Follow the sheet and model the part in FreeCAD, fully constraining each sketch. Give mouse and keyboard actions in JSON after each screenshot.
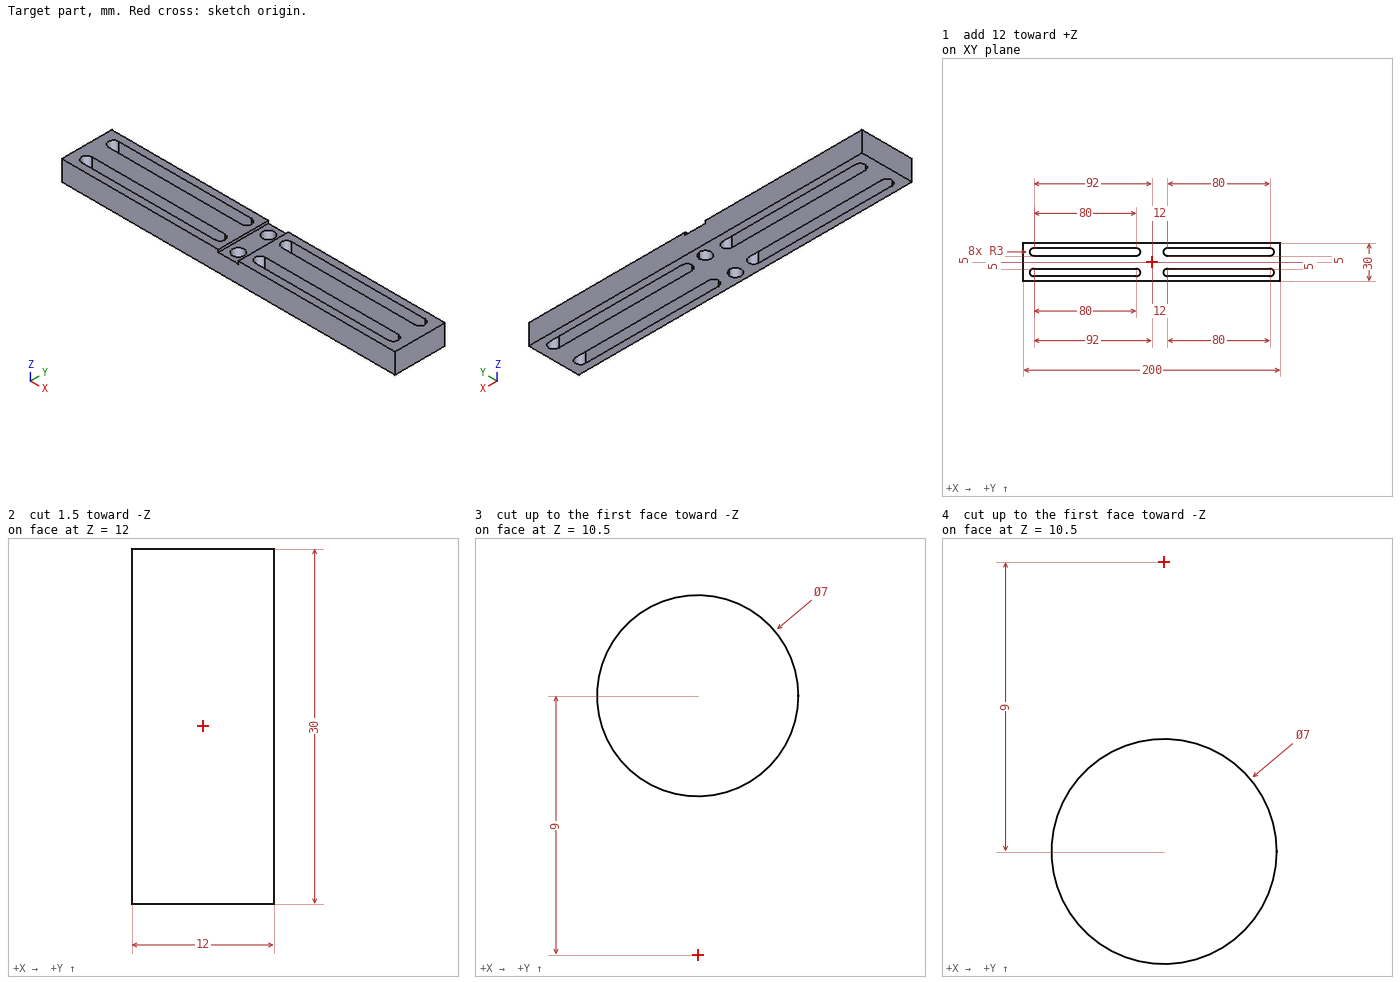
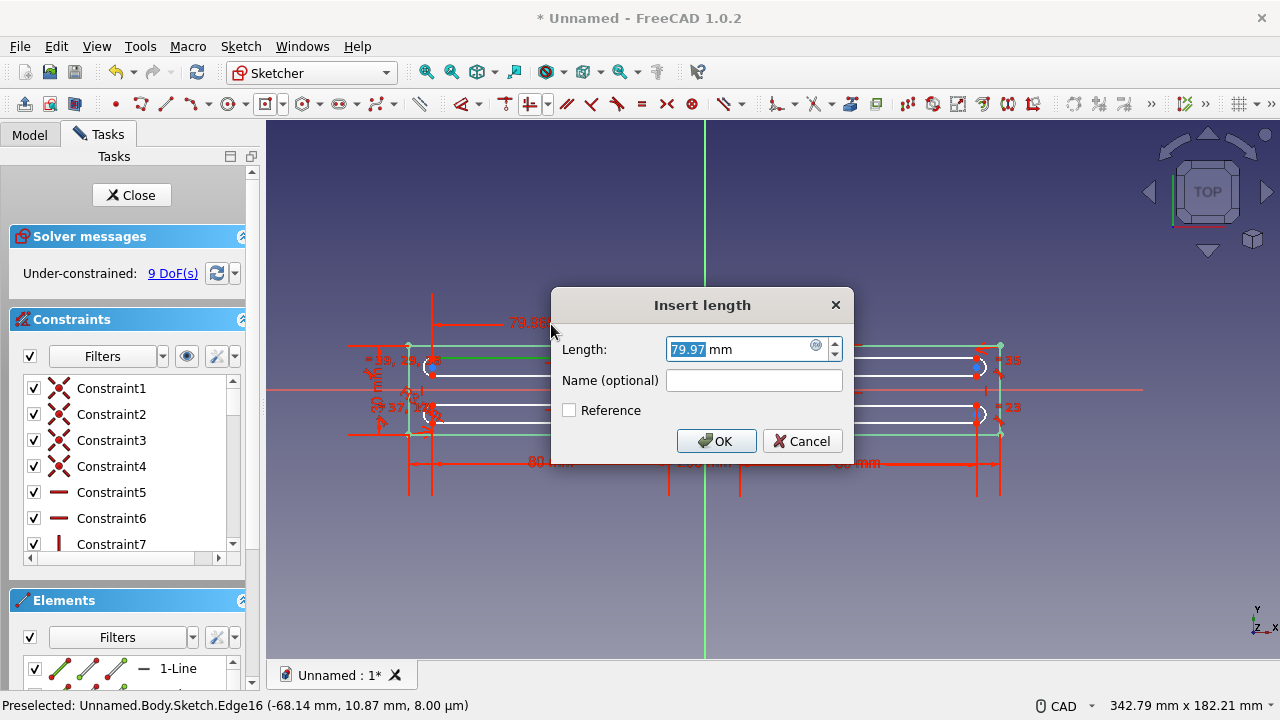
{"action": "type", "text": "80"}
{"action": "key", "text": "Return"}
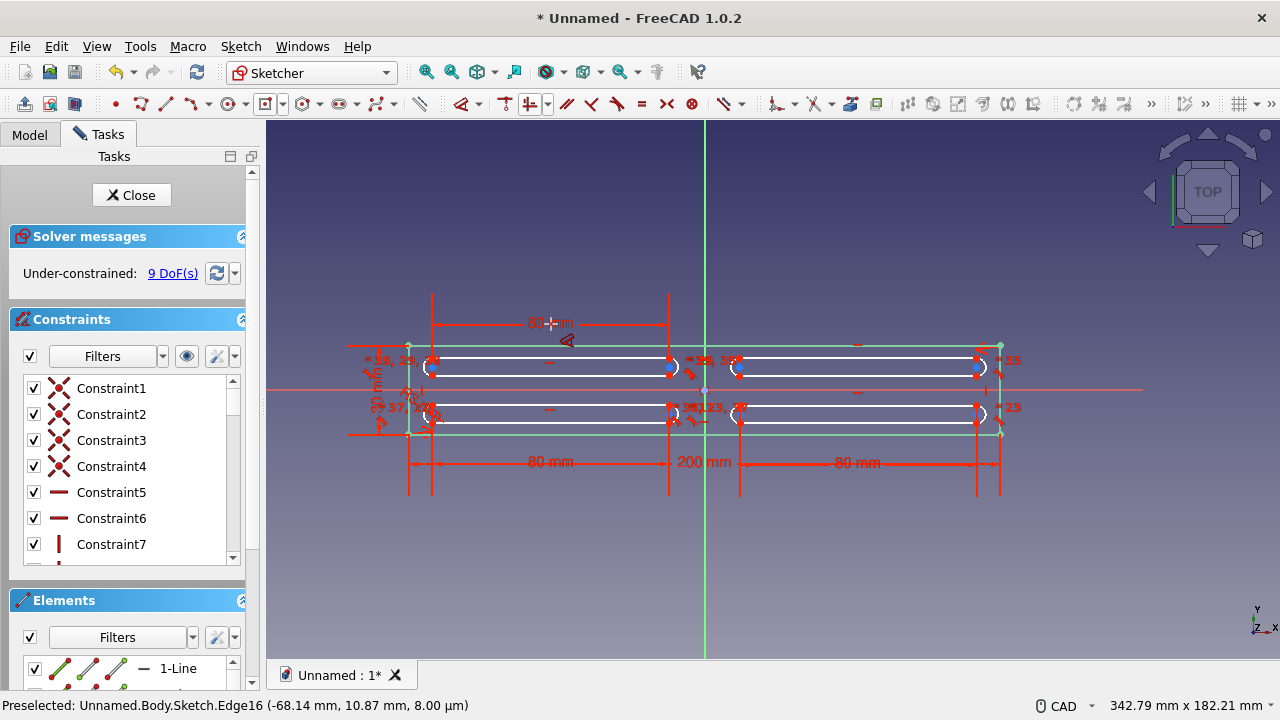
{"action": "left_click", "coordinate": [811, 358]}
{"action": "left_click", "coordinate": [858, 324]}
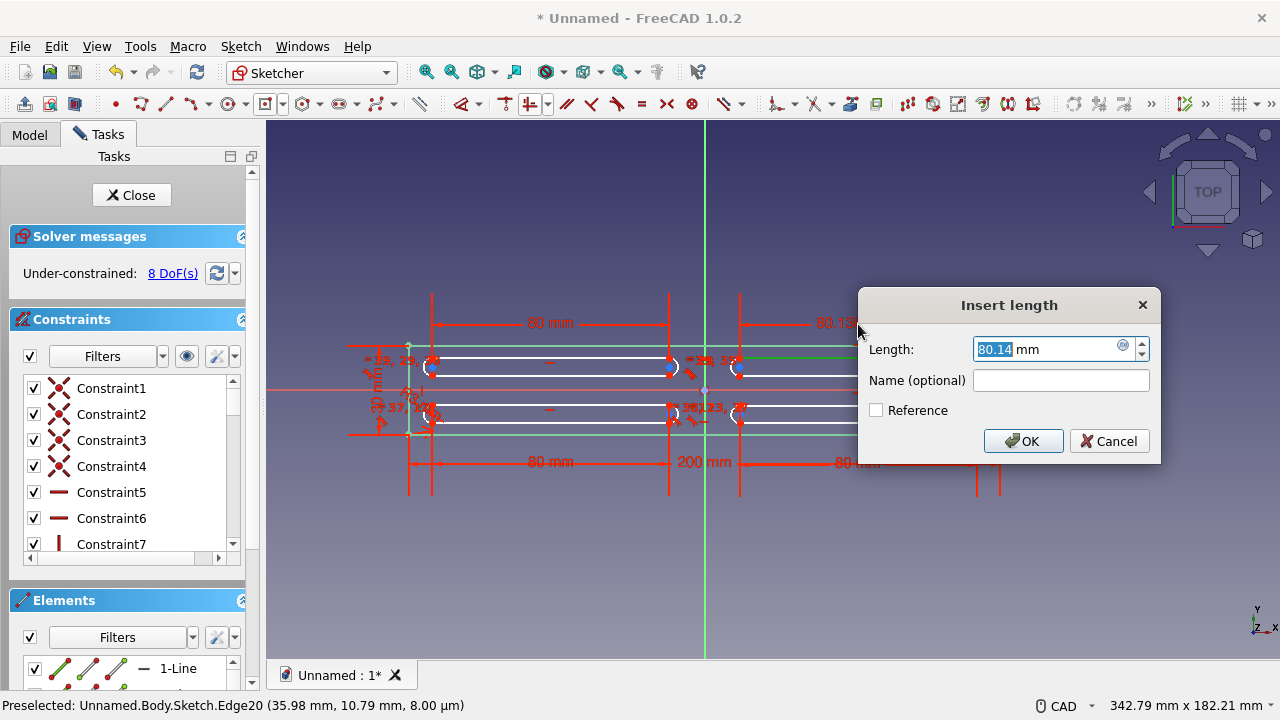
{"action": "type", "text": "80"}
{"action": "key", "text": "Return"}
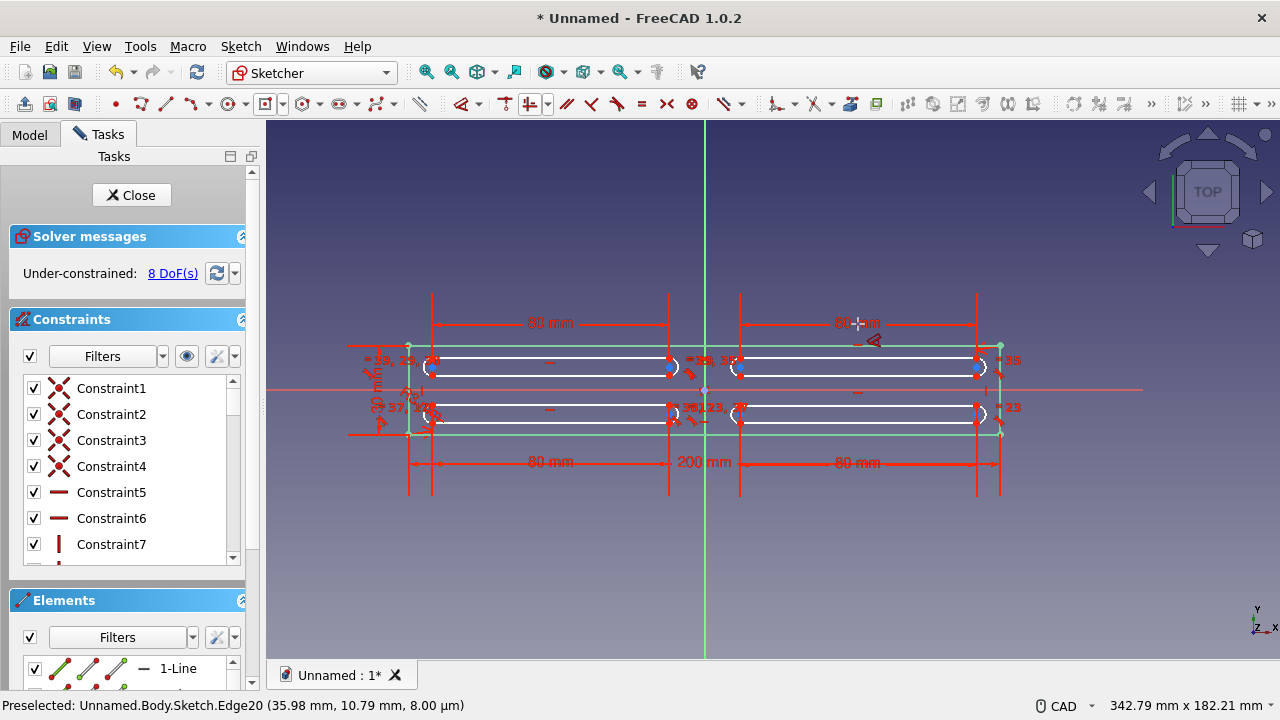
{"action": "scroll", "coordinate": [432, 405], "scroll_direction": "up", "scroll_amount": 5}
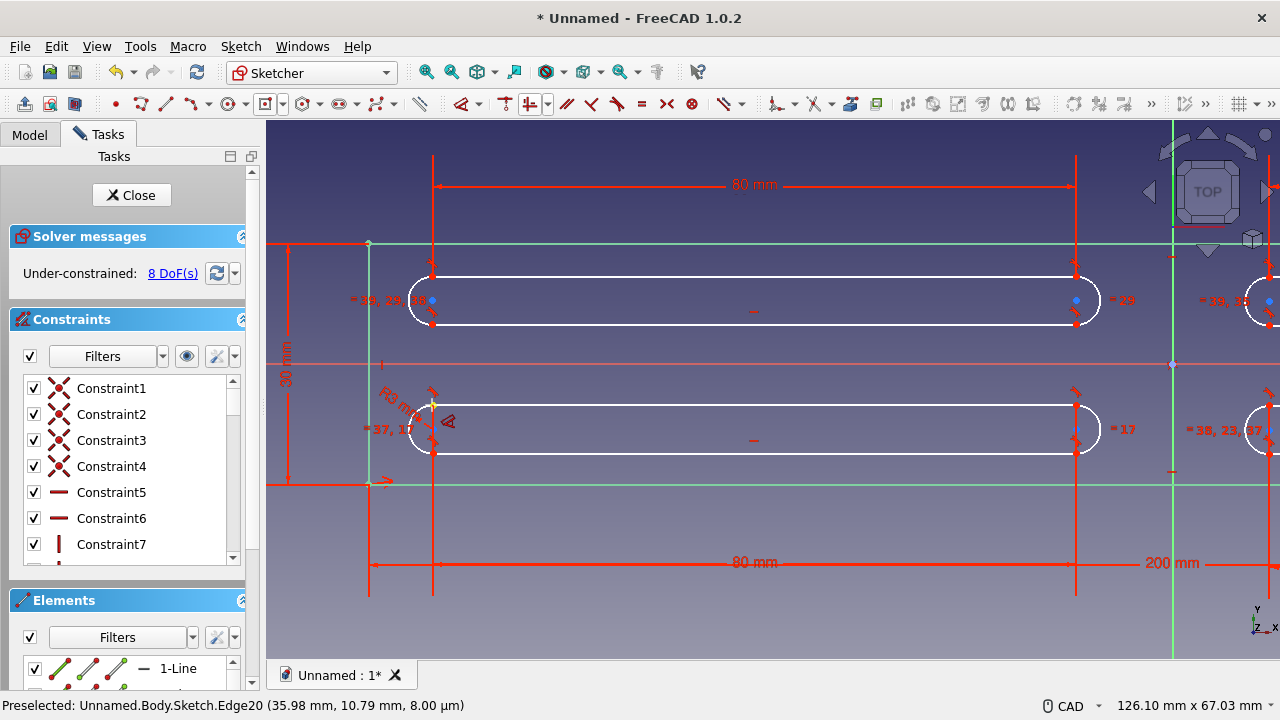
{"action": "left_click", "coordinate": [433, 405]}
{"action": "left_click", "coordinate": [399, 385]}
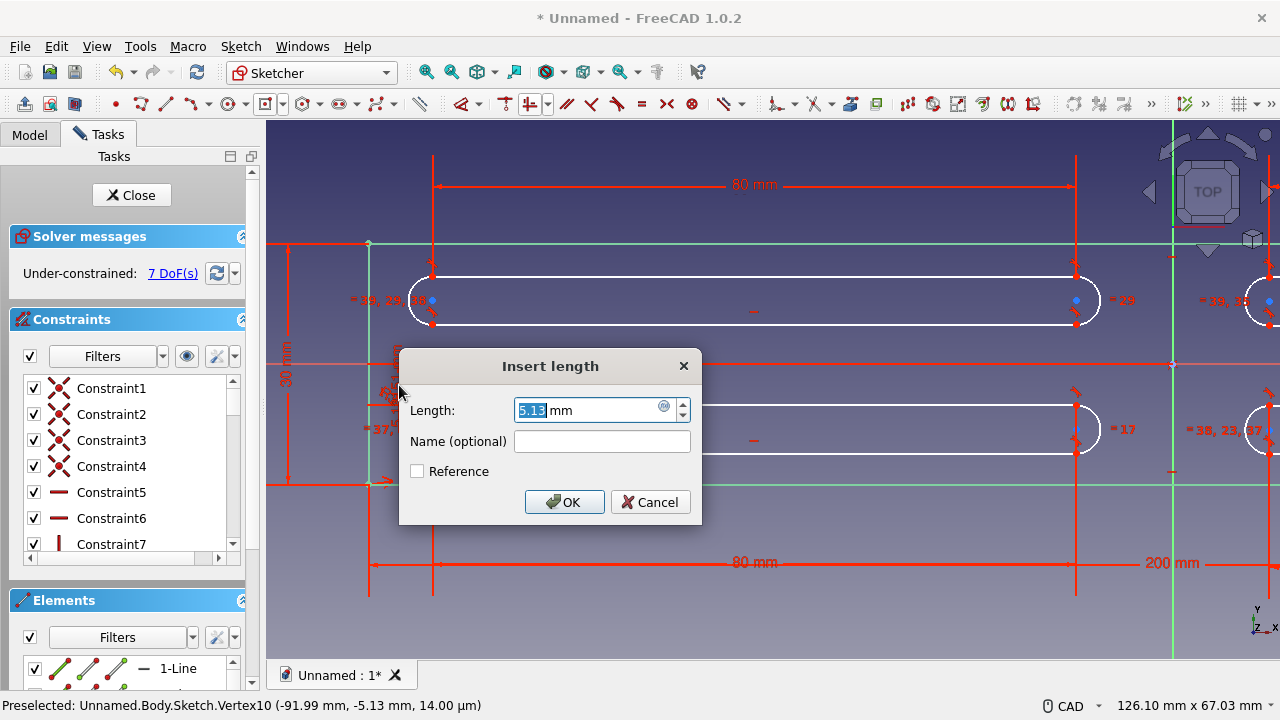
{"action": "type", "text": "5"}
{"action": "key", "text": "Return"}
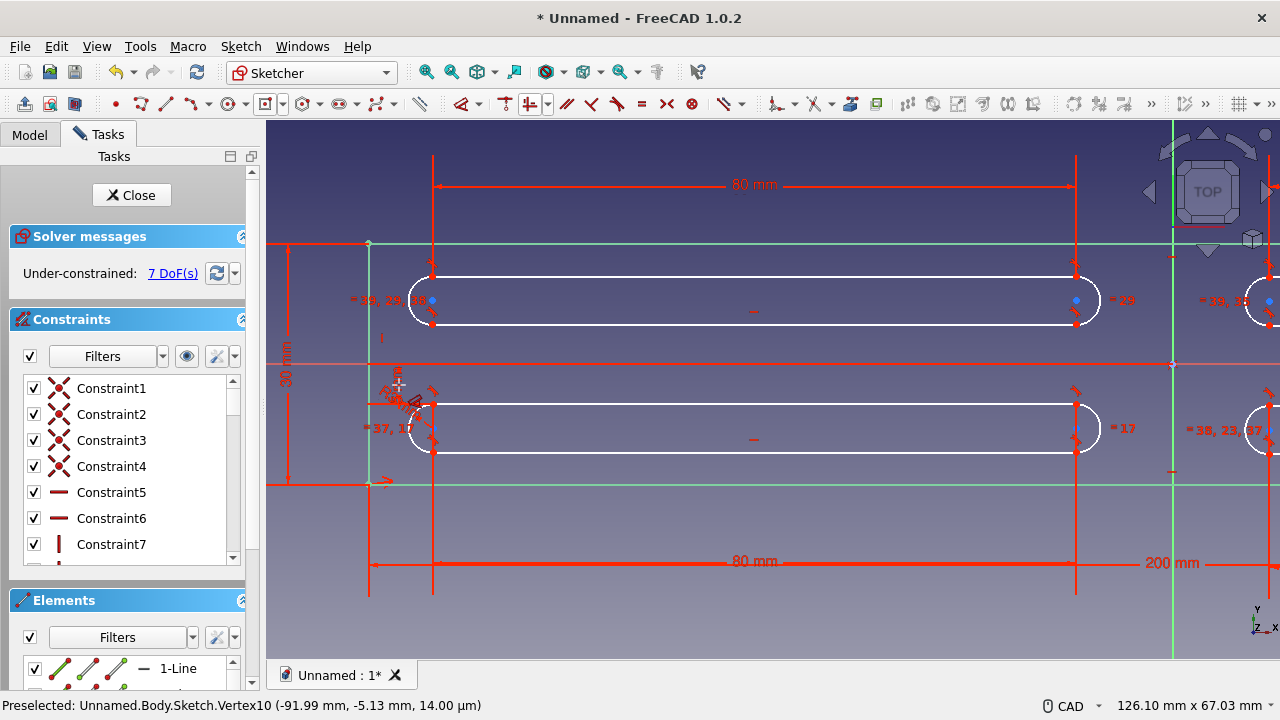
{"action": "scroll", "coordinate": [432, 404], "scroll_direction": "down", "scroll_amount": 5}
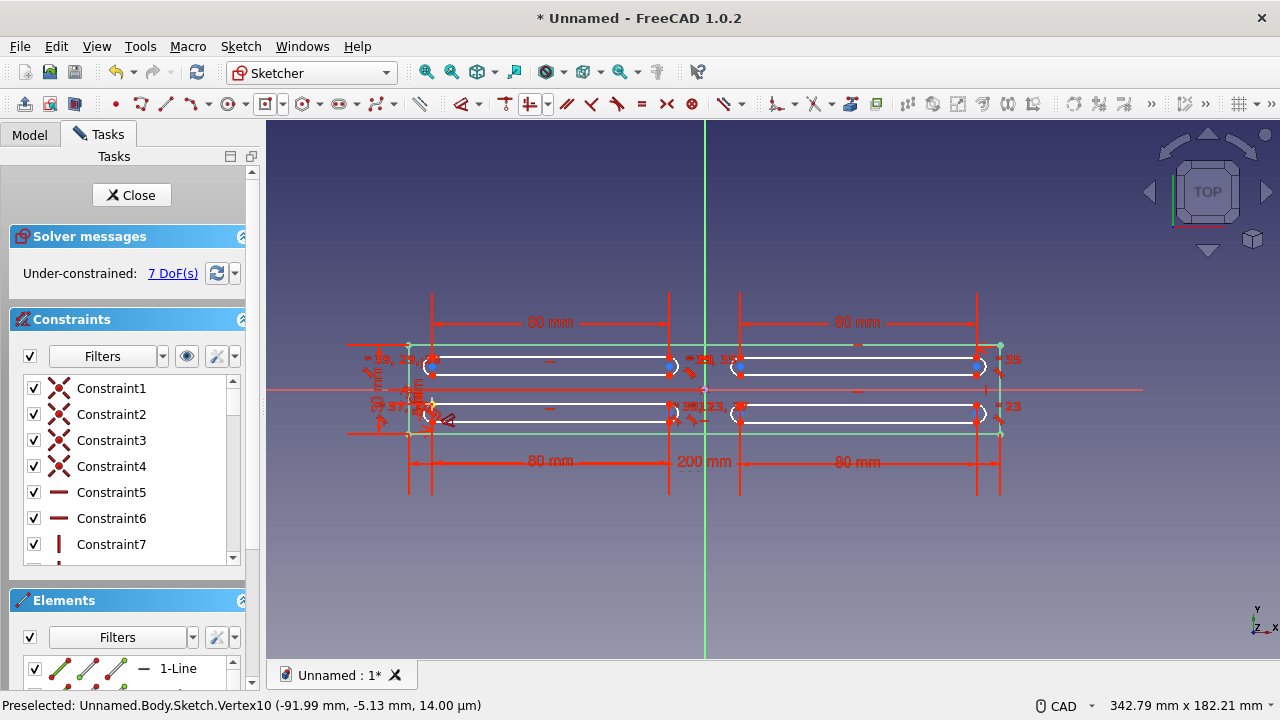
{"action": "scroll", "coordinate": [740, 405], "scroll_direction": "up", "scroll_amount": 5}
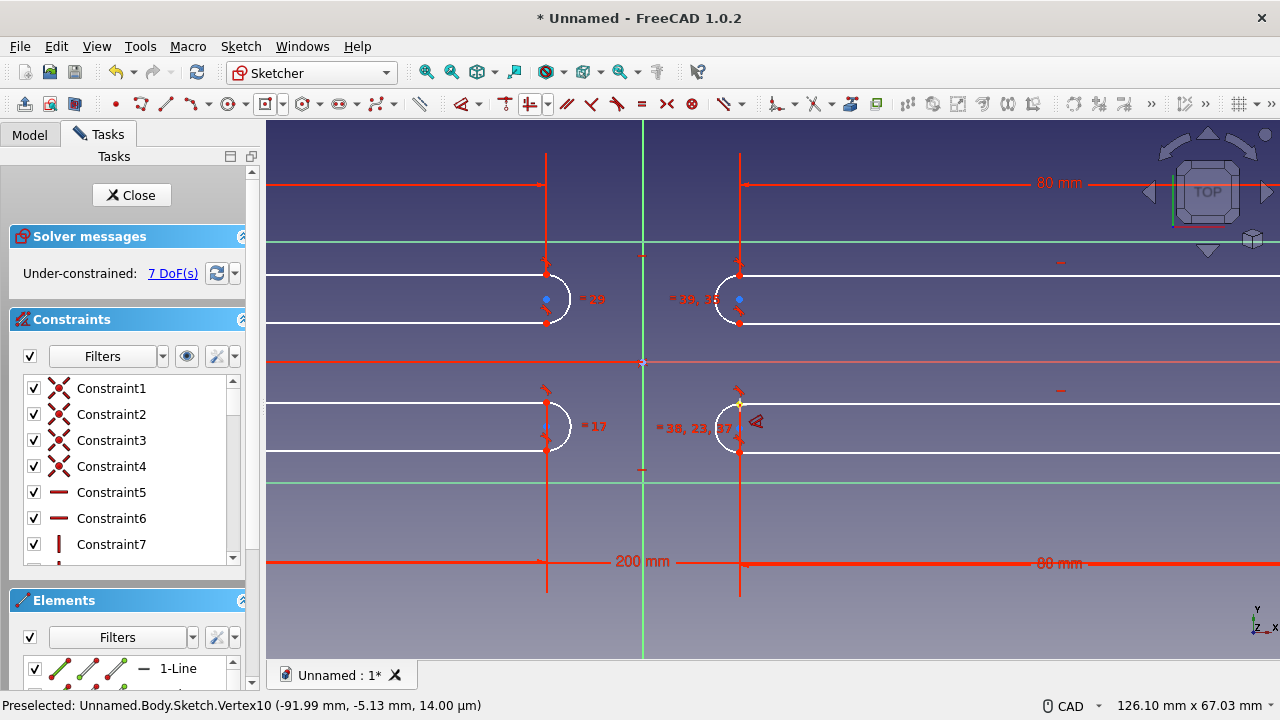
{"action": "left_click", "coordinate": [740, 404]}
{"action": "left_click", "coordinate": [774, 383]}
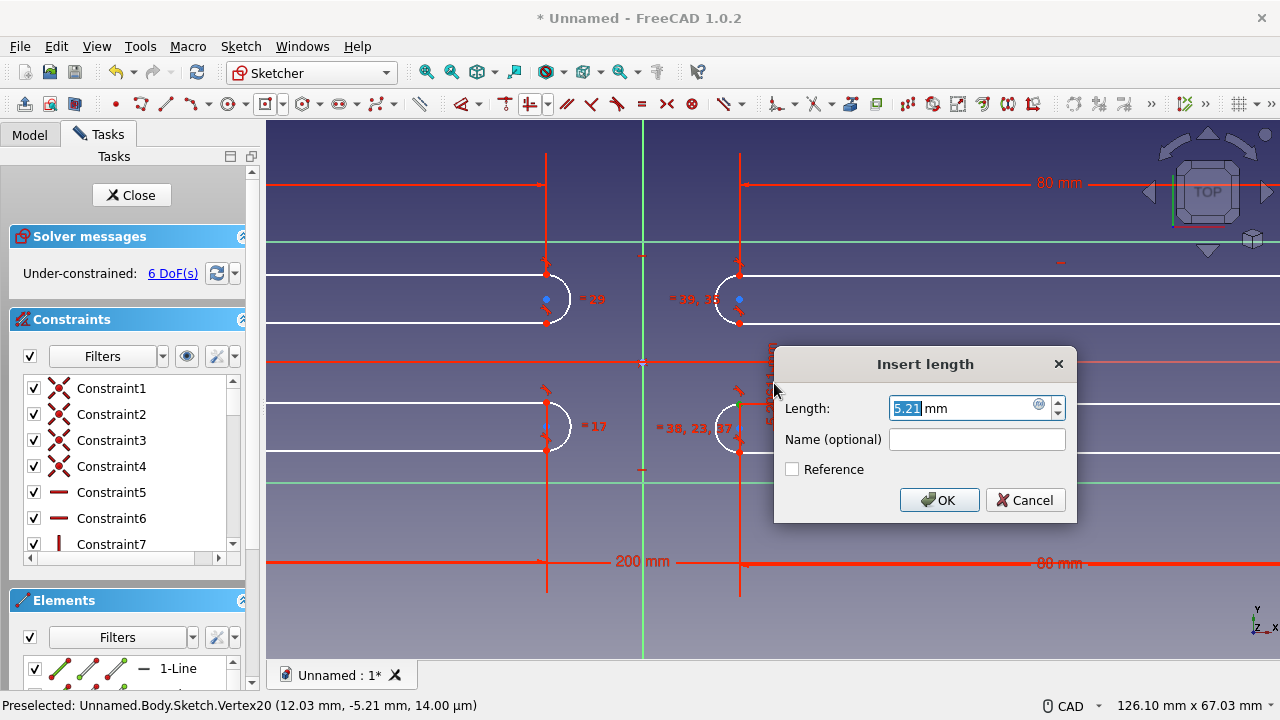
{"action": "type", "text": "5"}
{"action": "key", "text": "Return"}